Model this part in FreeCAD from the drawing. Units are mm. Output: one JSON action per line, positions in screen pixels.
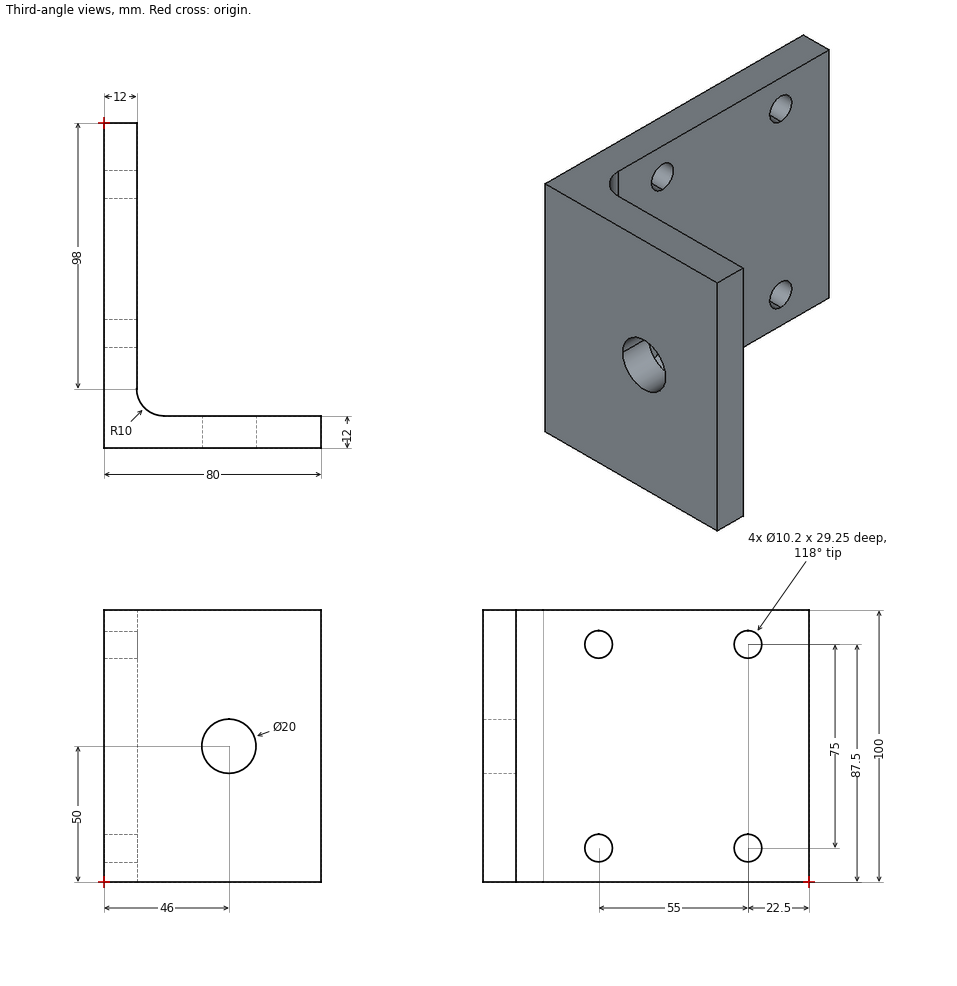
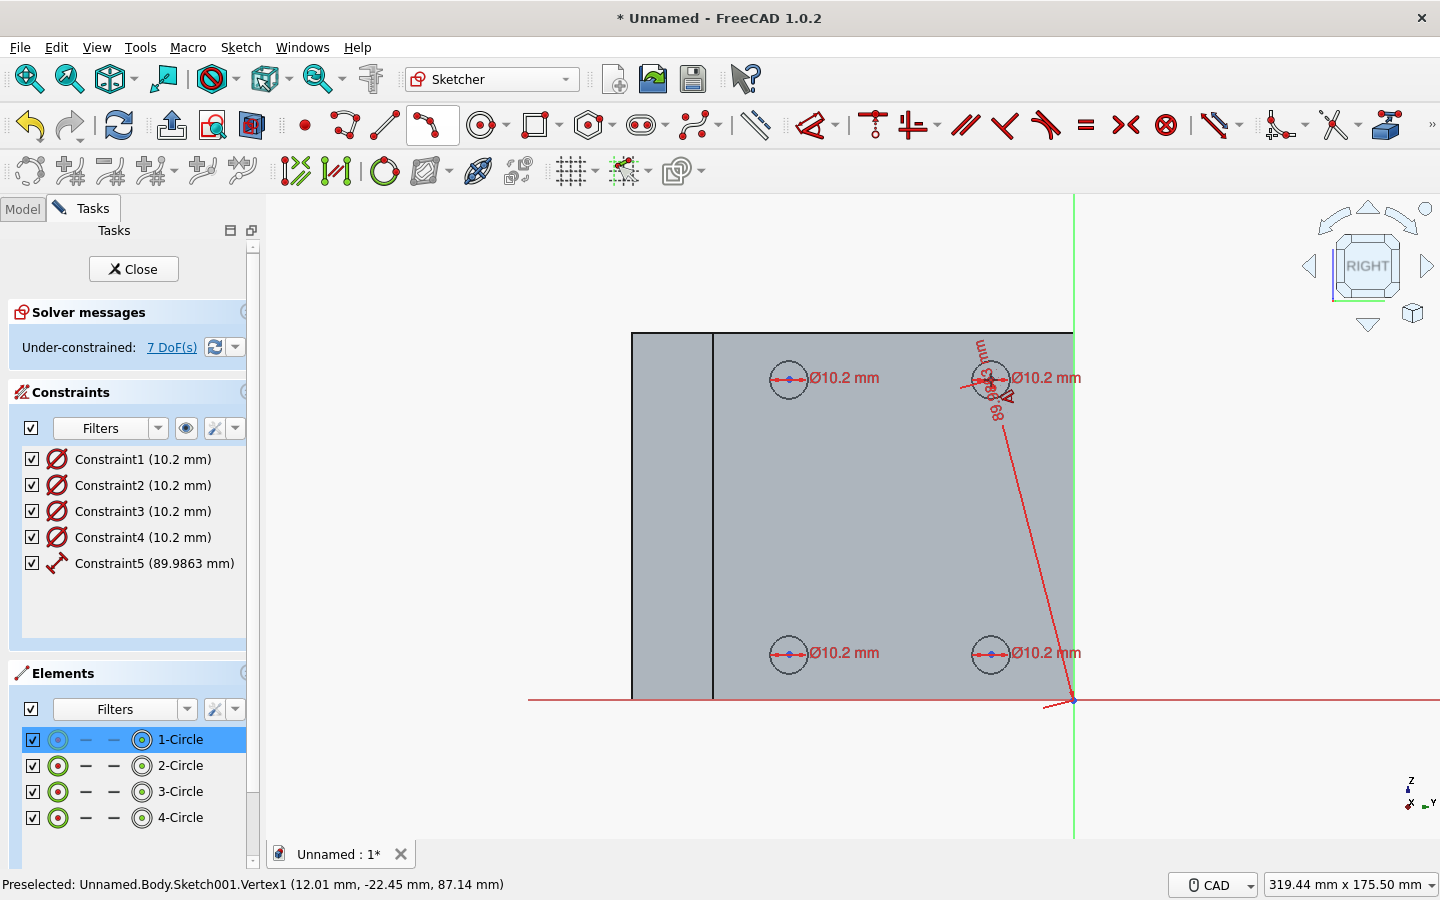
{"action": "left_click", "coordinate": [991, 655]}
{"action": "left_click", "coordinate": [1025, 518]}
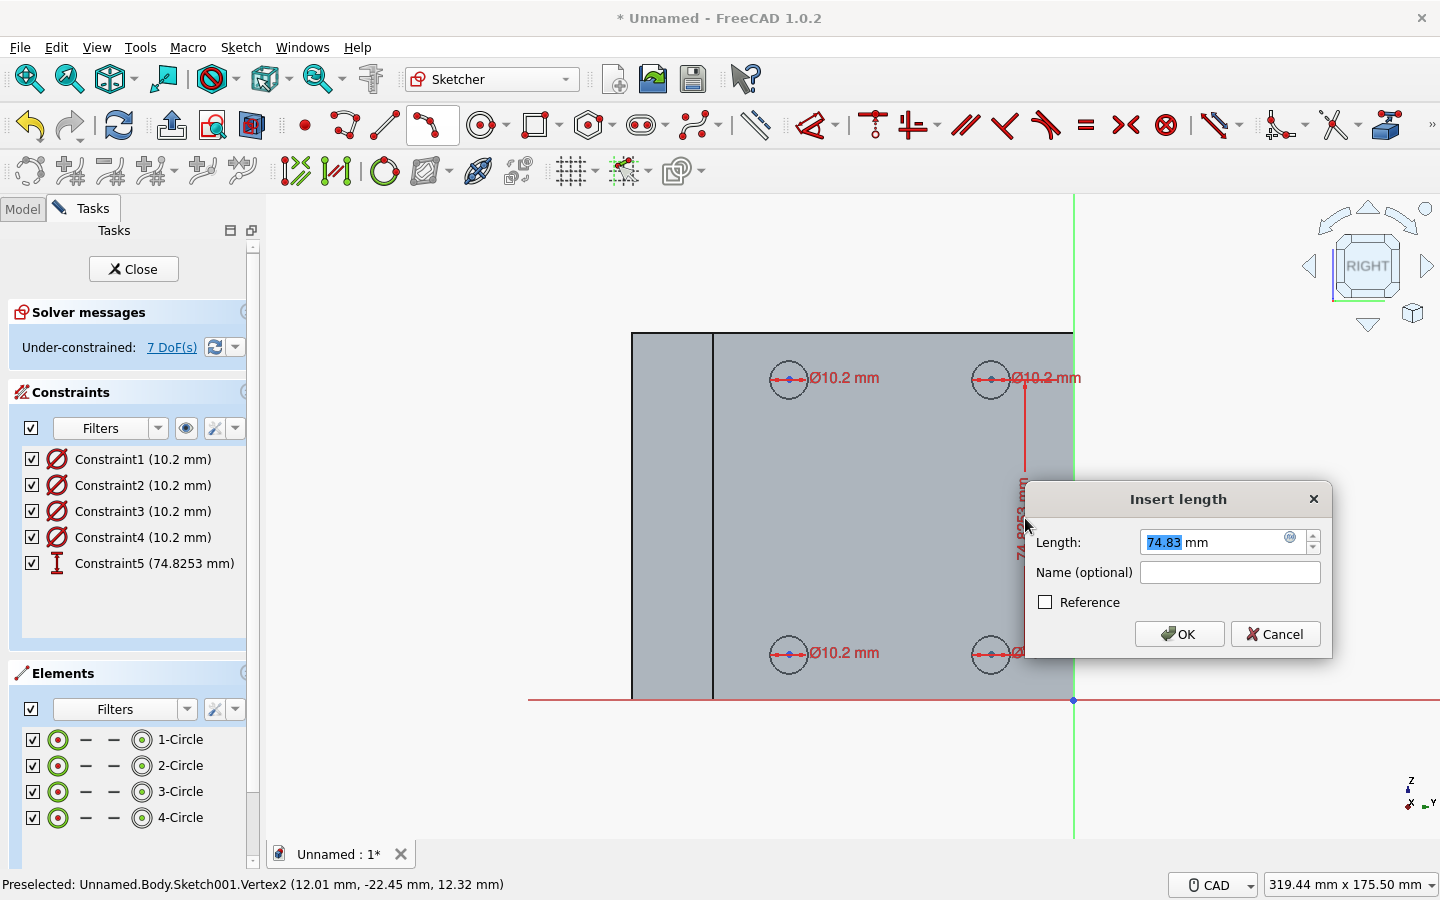
{"action": "type", "text": "75"}
{"action": "key", "text": "Return"}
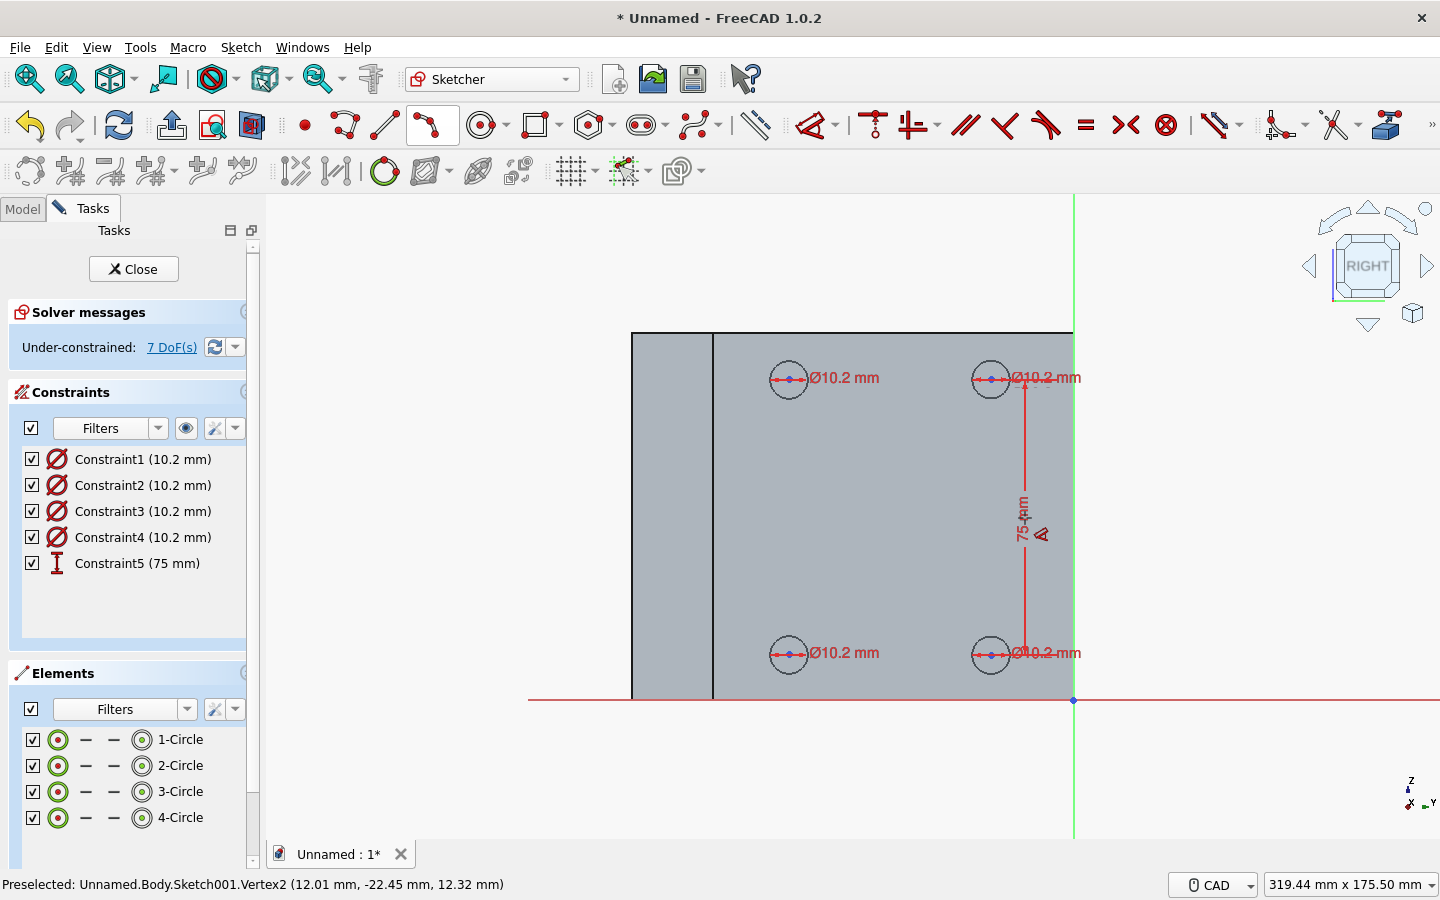
{"action": "left_click", "coordinate": [991, 655]}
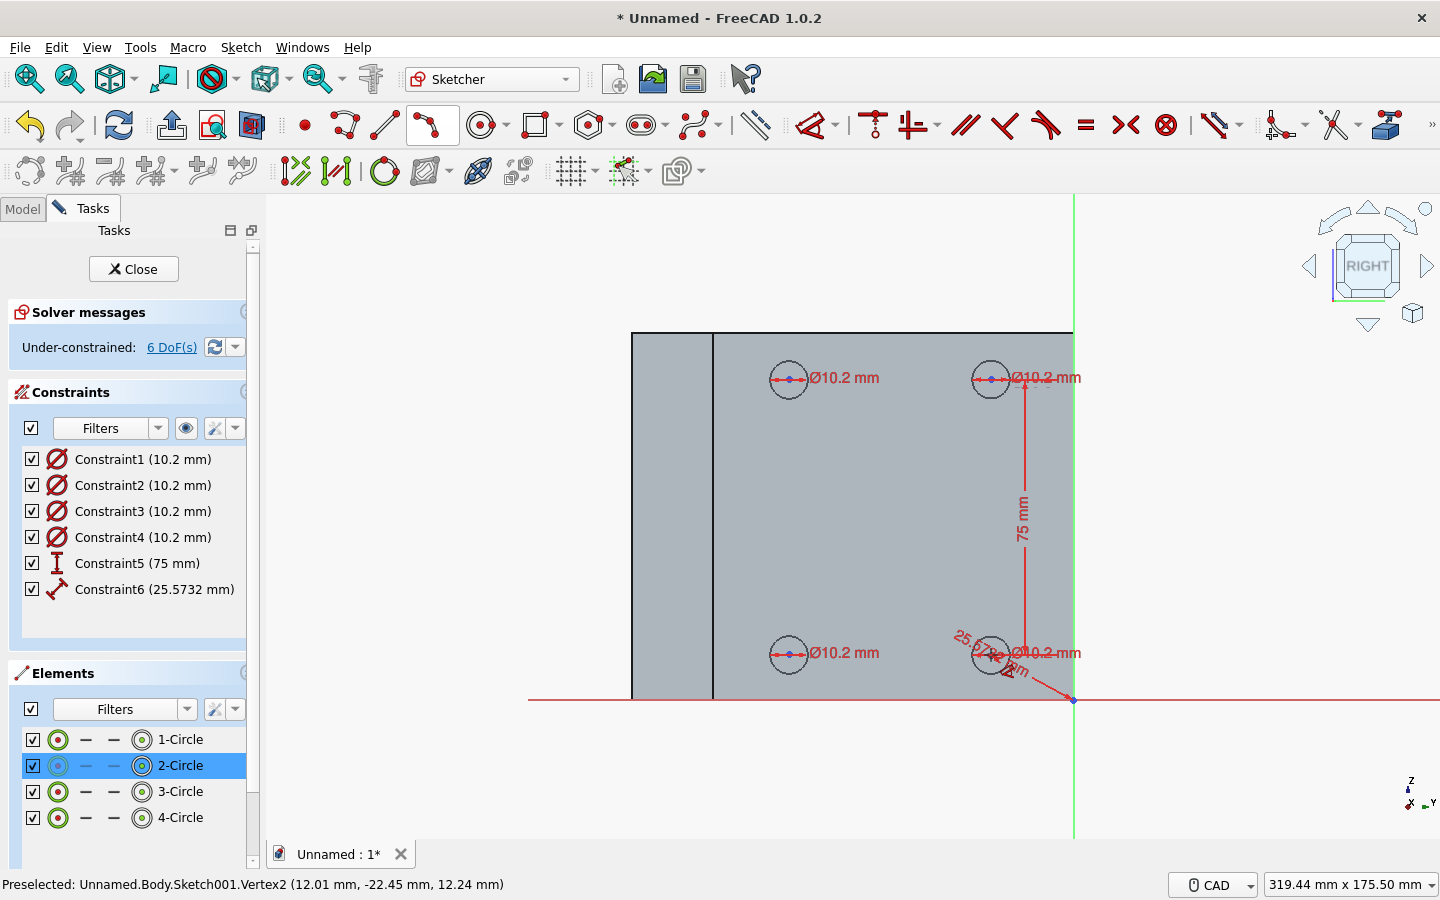
{"action": "left_click", "coordinate": [789, 655]}
{"action": "left_click", "coordinate": [890, 621]}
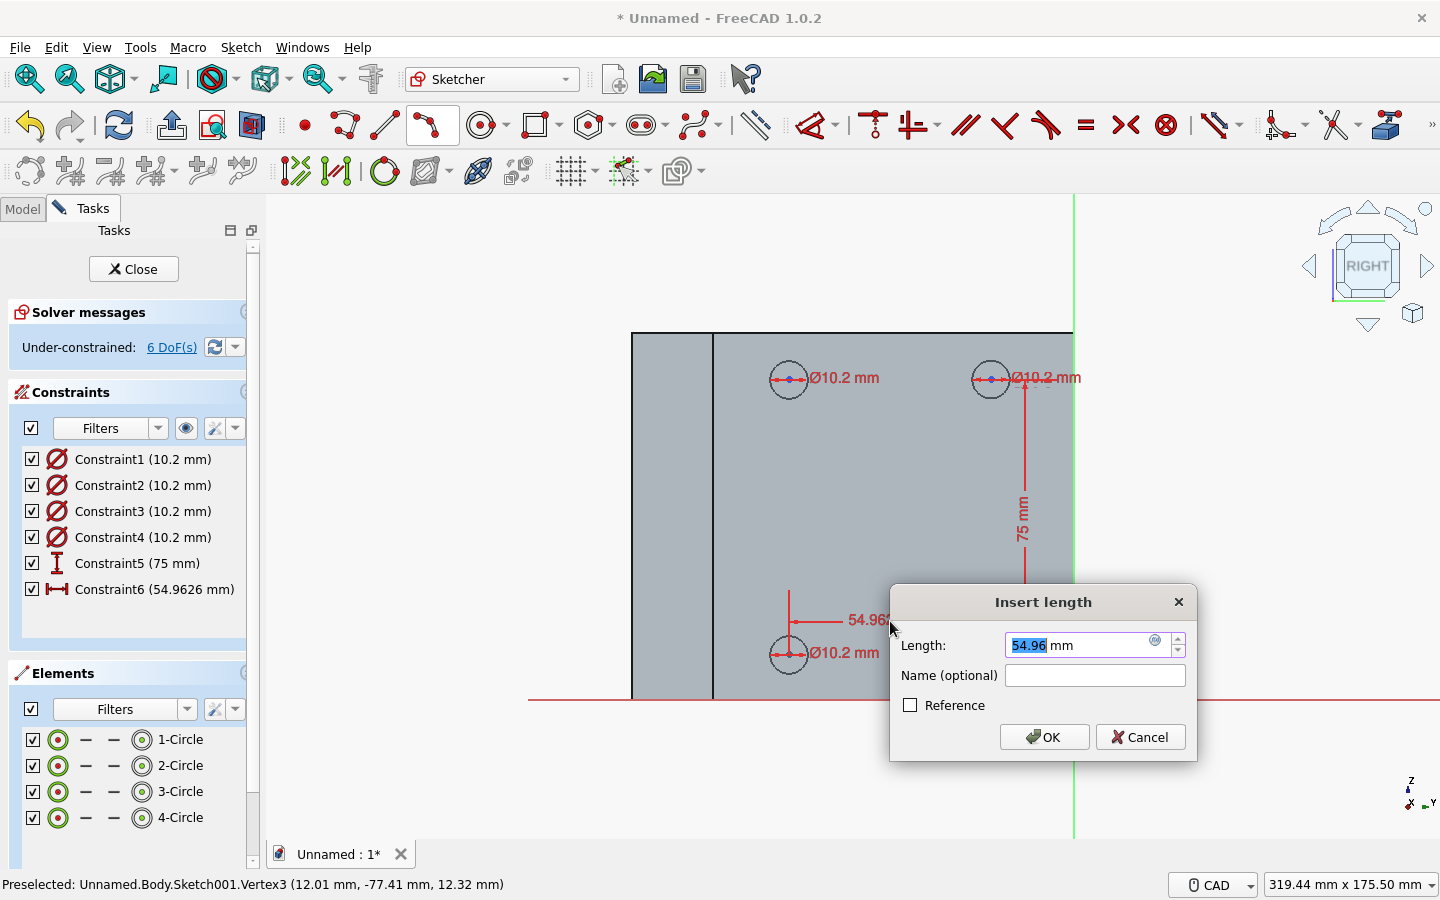
{"action": "type", "text": "55"}
{"action": "key", "text": "Return"}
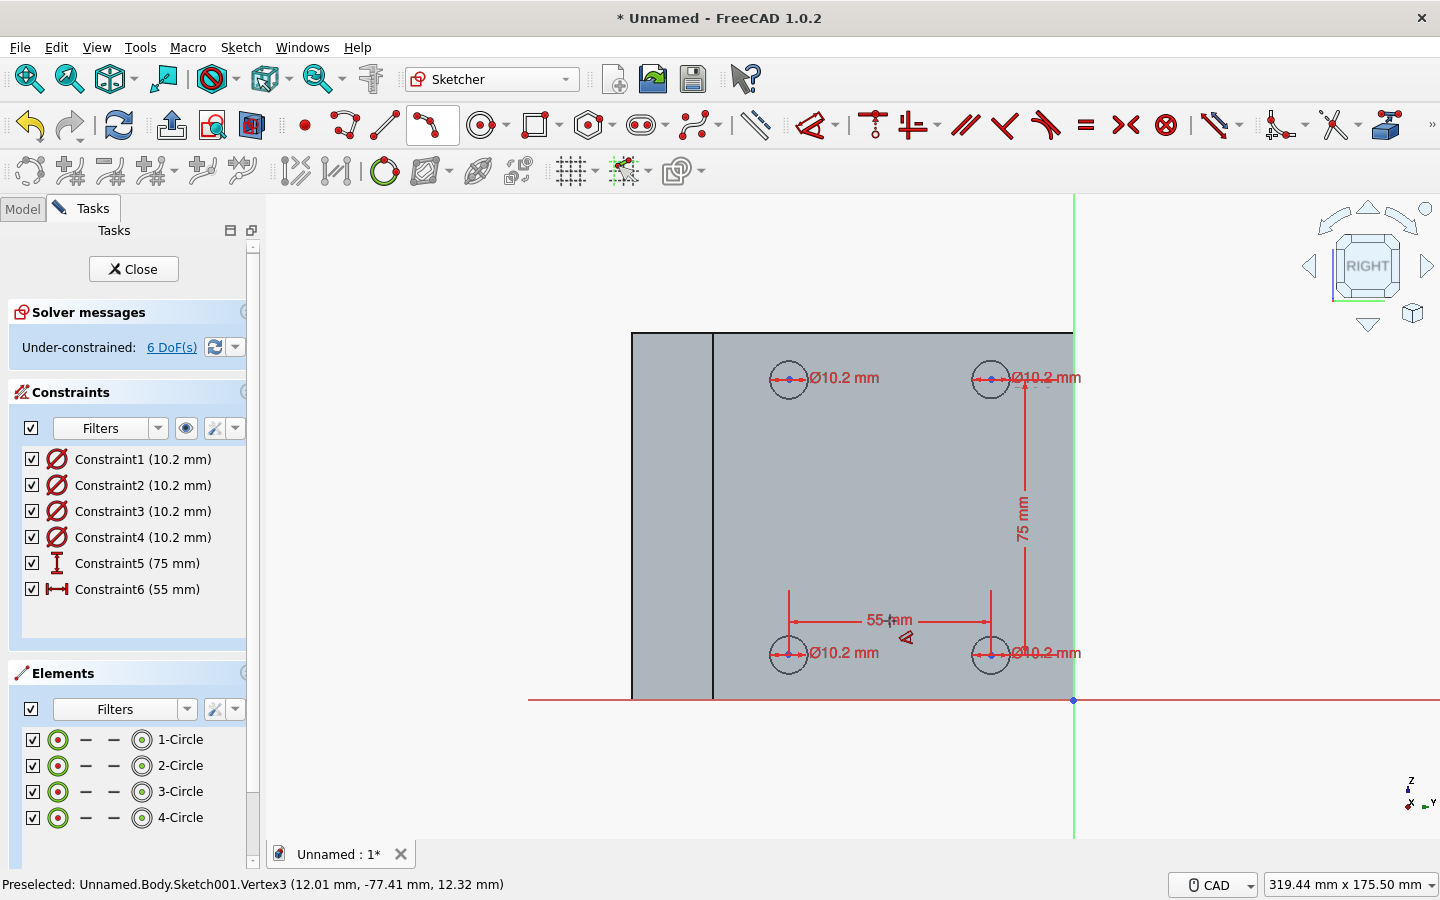
{"action": "left_click", "coordinate": [991, 380]}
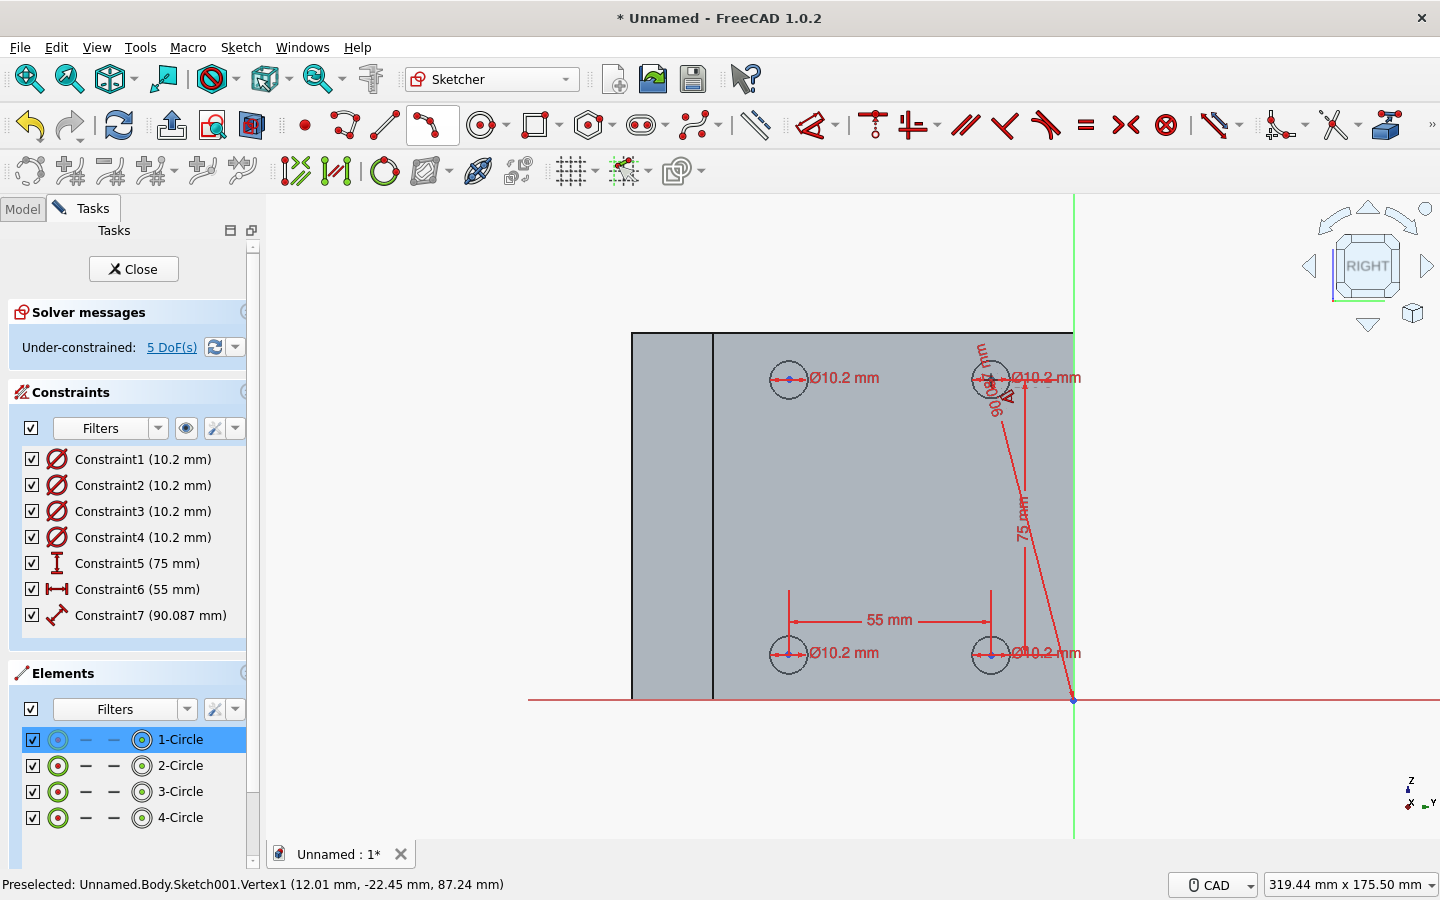
{"action": "left_click", "coordinate": [789, 655]}
{"action": "left_click", "coordinate": [890, 346]}